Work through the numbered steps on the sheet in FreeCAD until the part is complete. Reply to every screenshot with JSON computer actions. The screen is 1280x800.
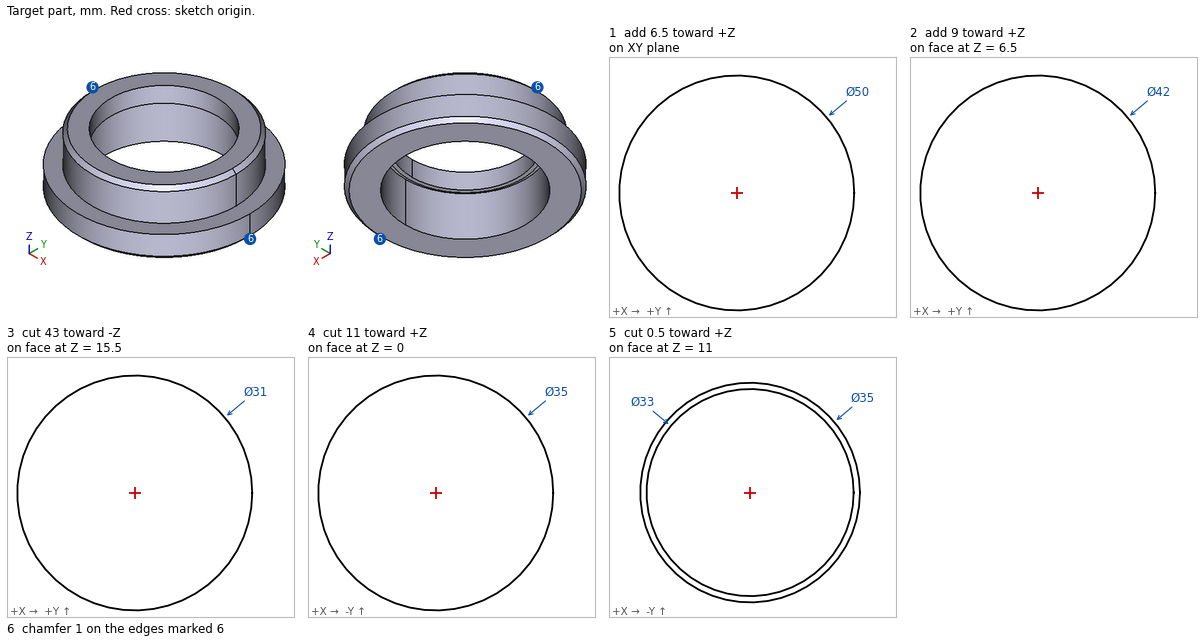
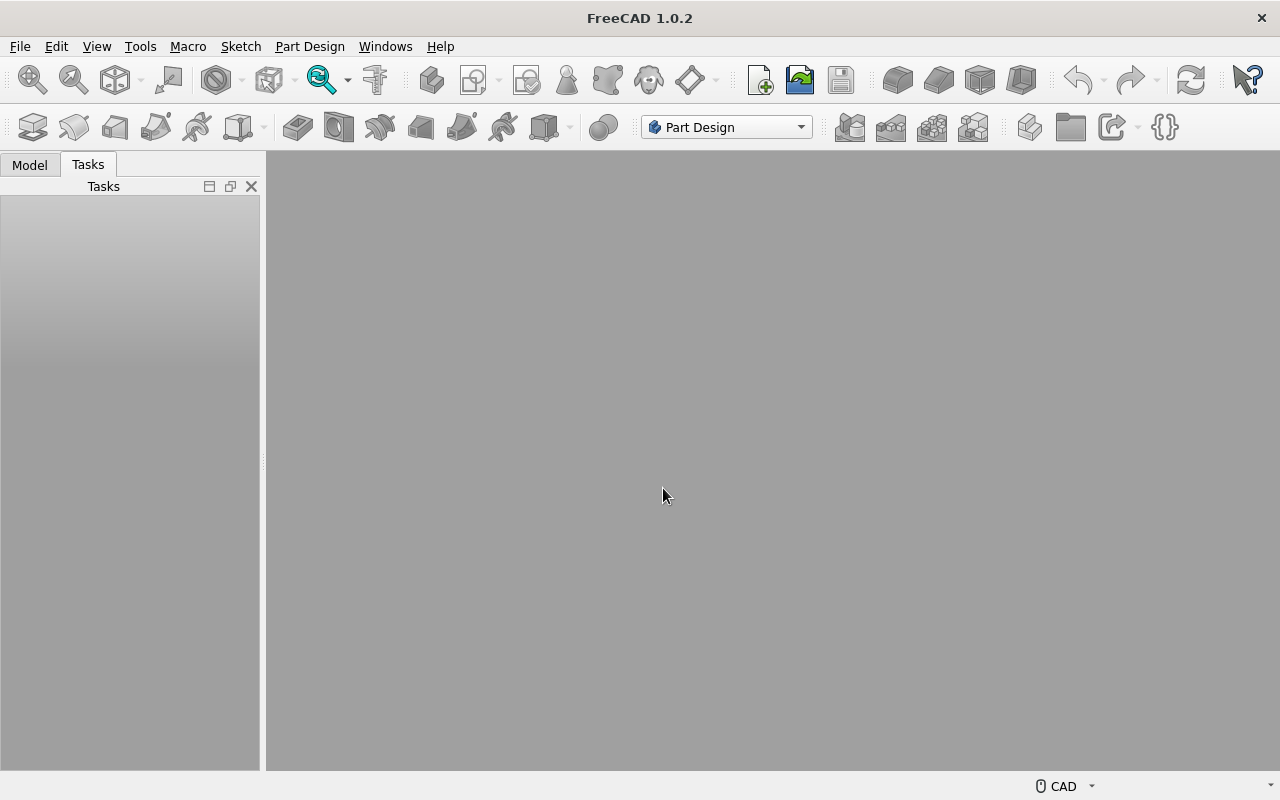
{"action": "left_click", "coordinate": [759, 80]}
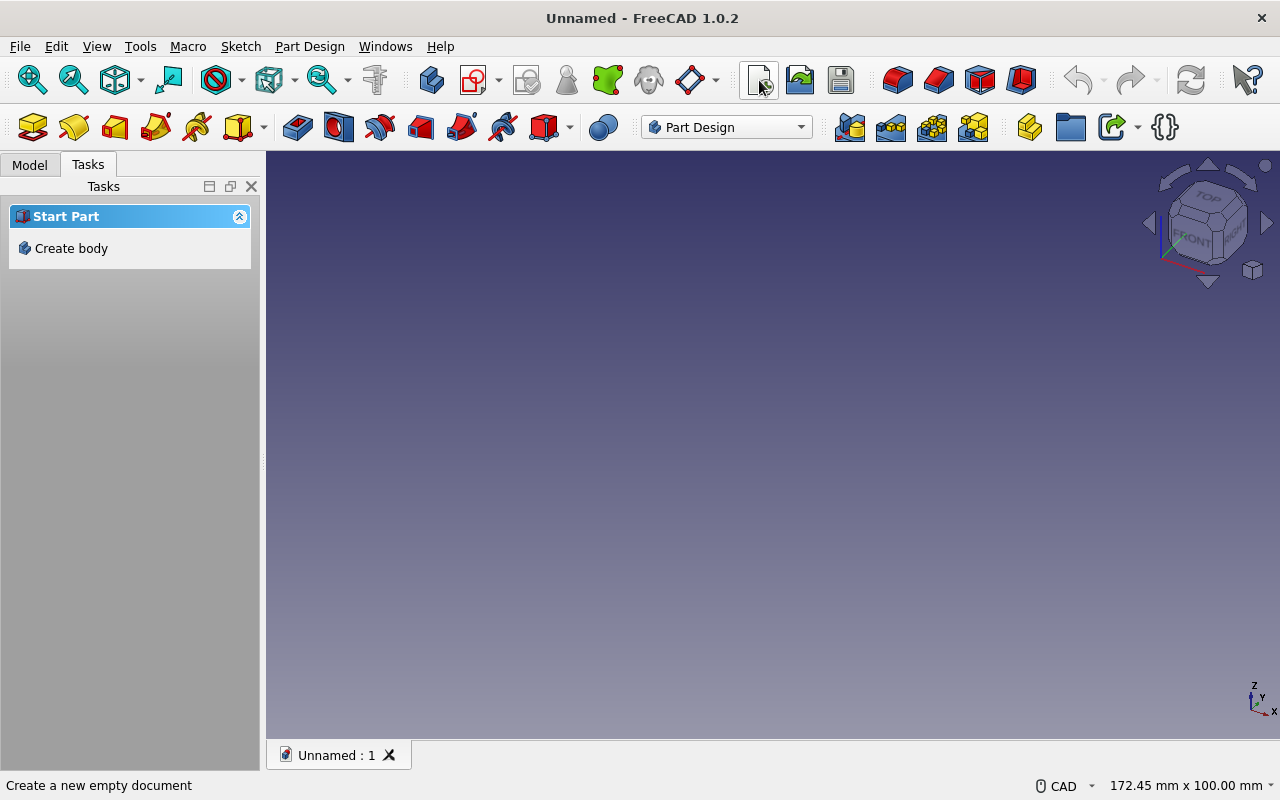
{"action": "left_click", "coordinate": [472, 80]}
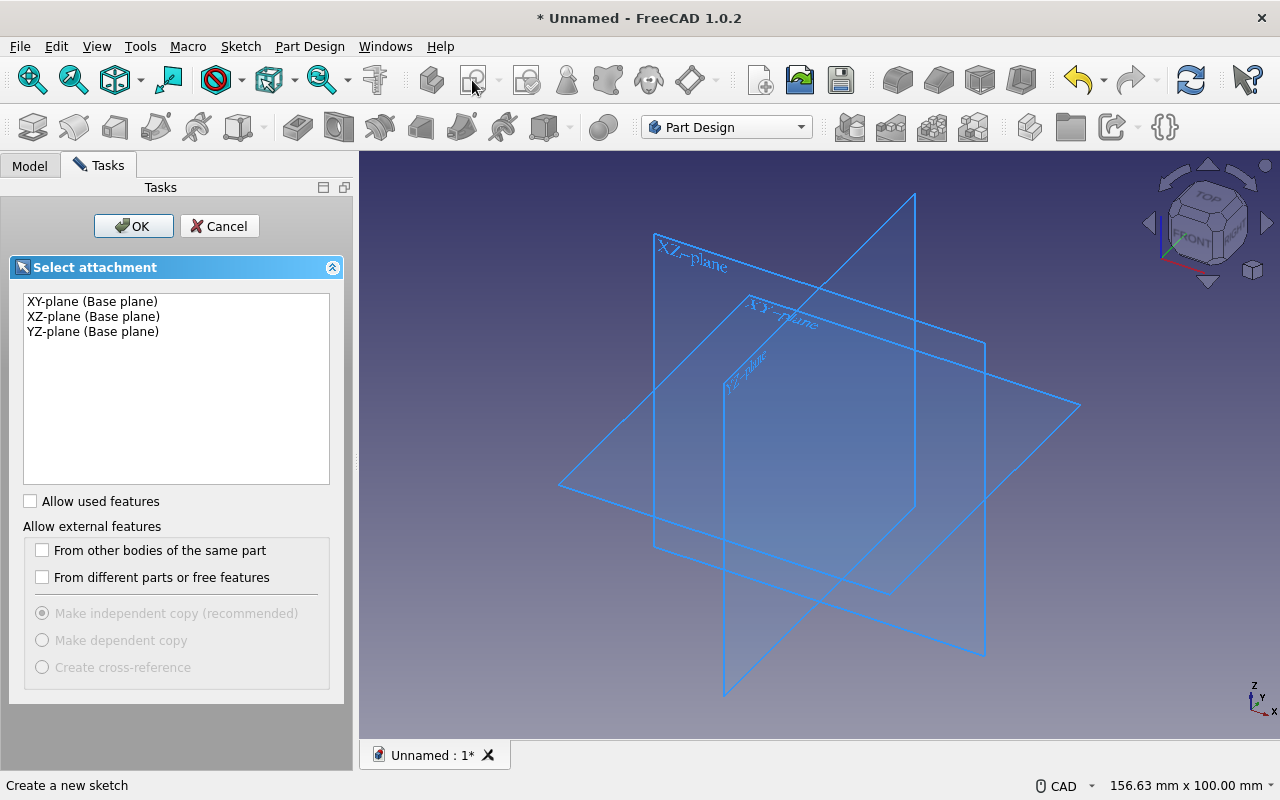
{"action": "left_click", "coordinate": [84, 302]}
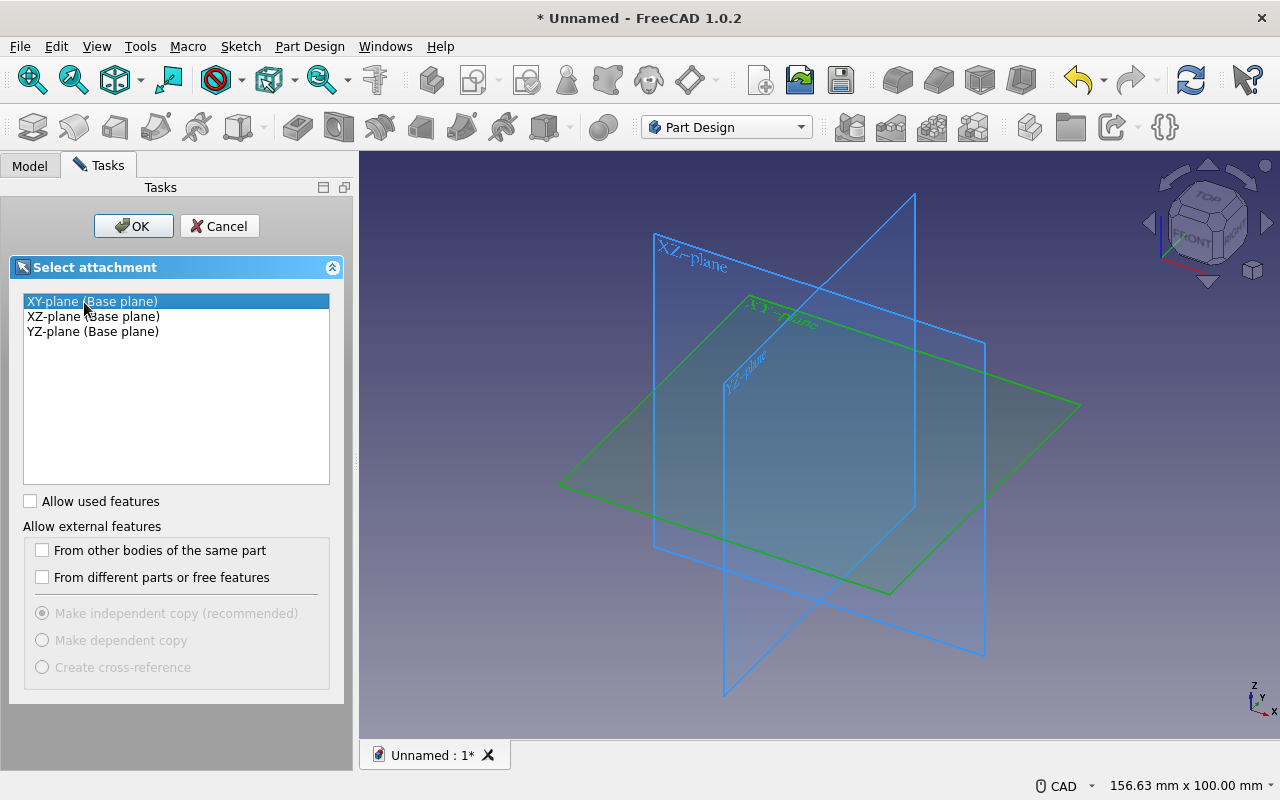
{"action": "left_click", "coordinate": [134, 226]}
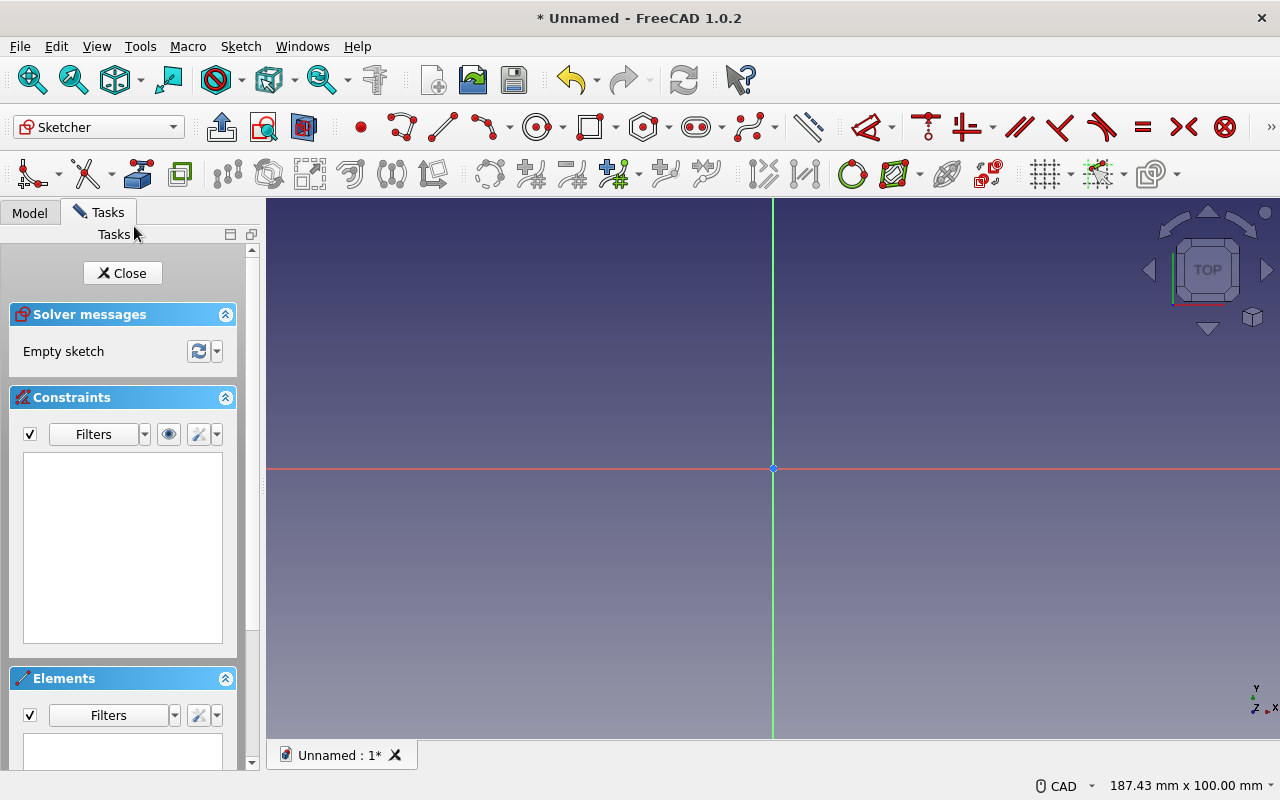
{"action": "left_click", "coordinate": [536, 128]}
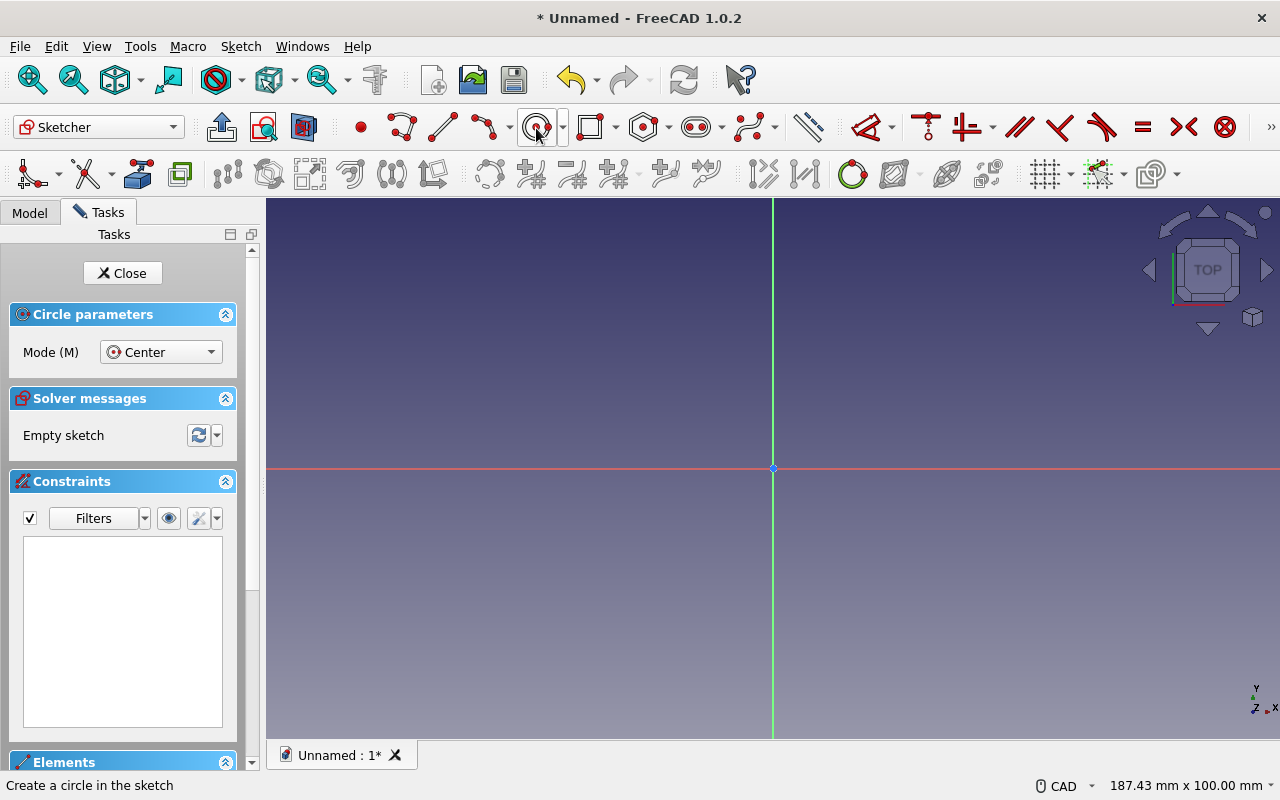
{"action": "left_click", "coordinate": [773, 468]}
{"action": "mouse_move", "coordinate": [869, 373]}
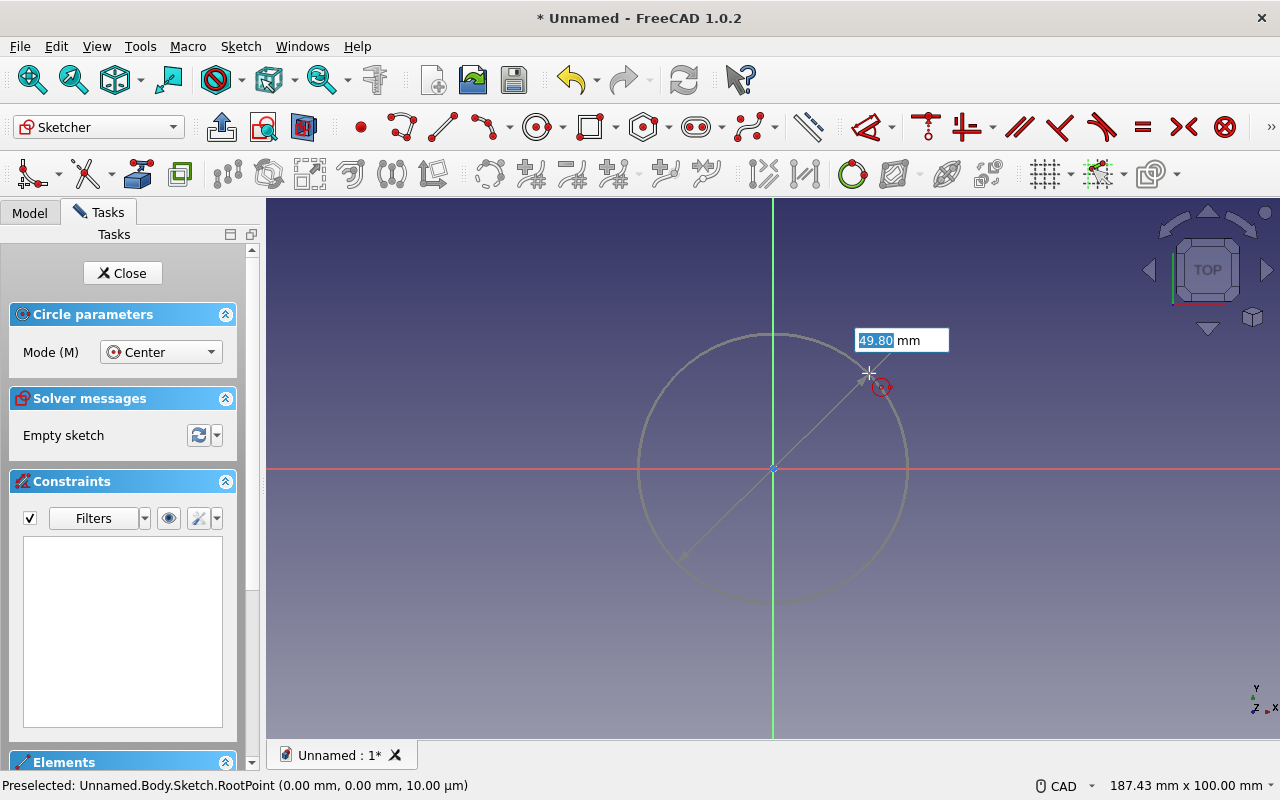
{"action": "type", "text": "50"}
{"action": "key", "text": "Return"}
{"action": "key", "text": "Escape"}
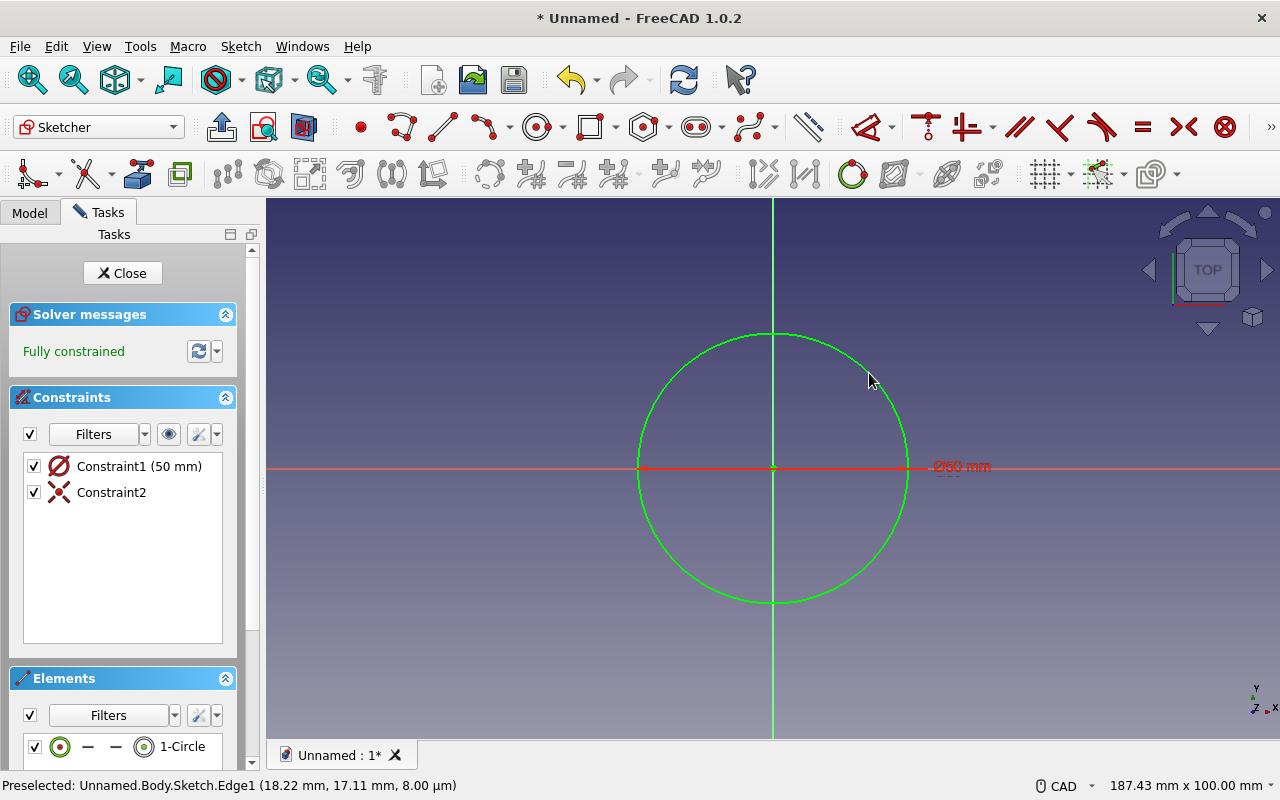
{"action": "left_click", "coordinate": [123, 273]}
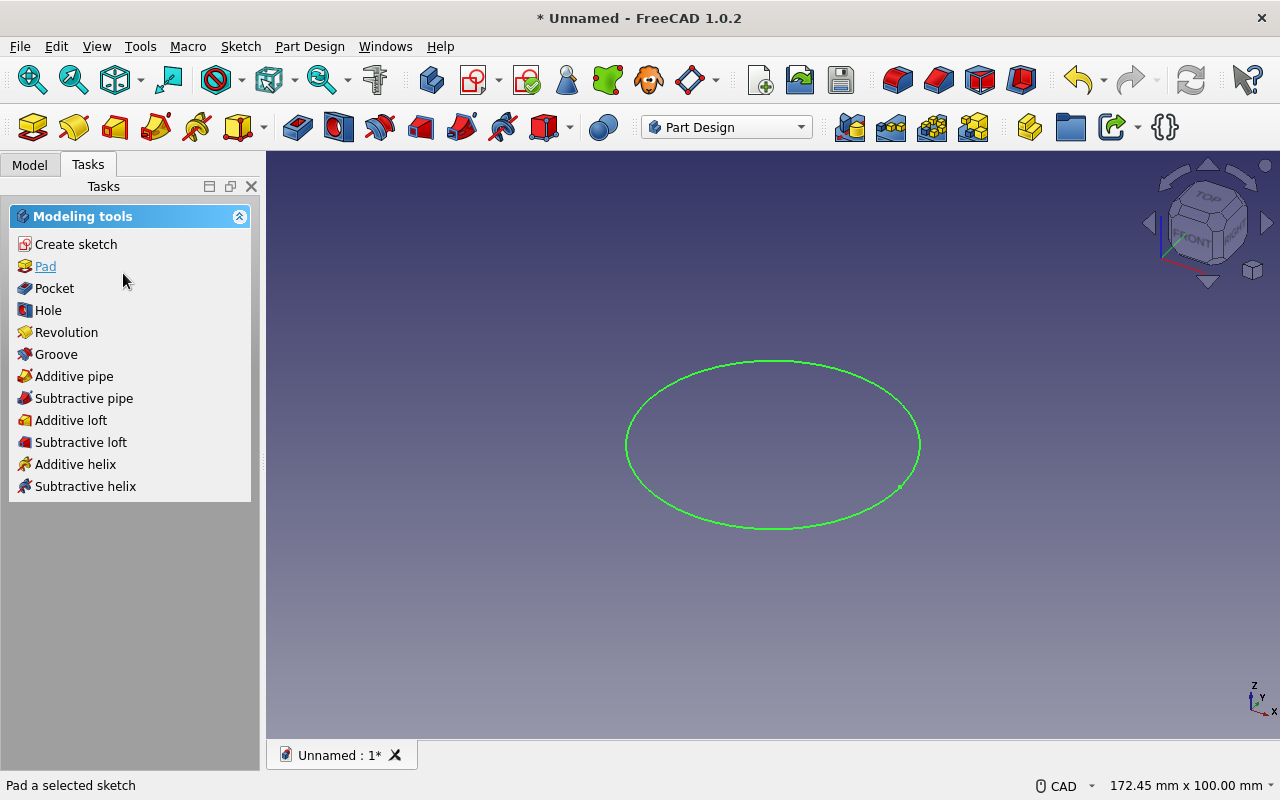
{"action": "left_click", "coordinate": [33, 128]}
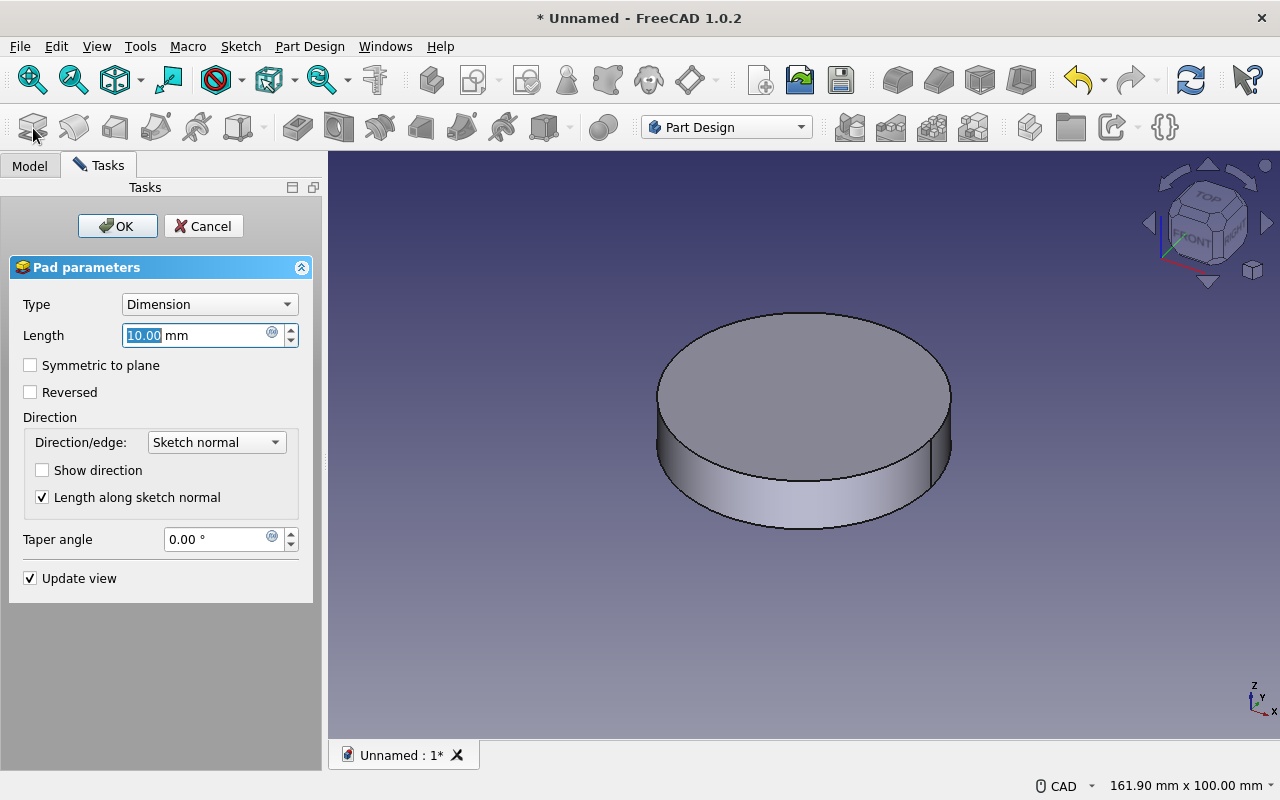
{"action": "type", "text": "6.5"}
{"action": "key", "text": "Tab"}